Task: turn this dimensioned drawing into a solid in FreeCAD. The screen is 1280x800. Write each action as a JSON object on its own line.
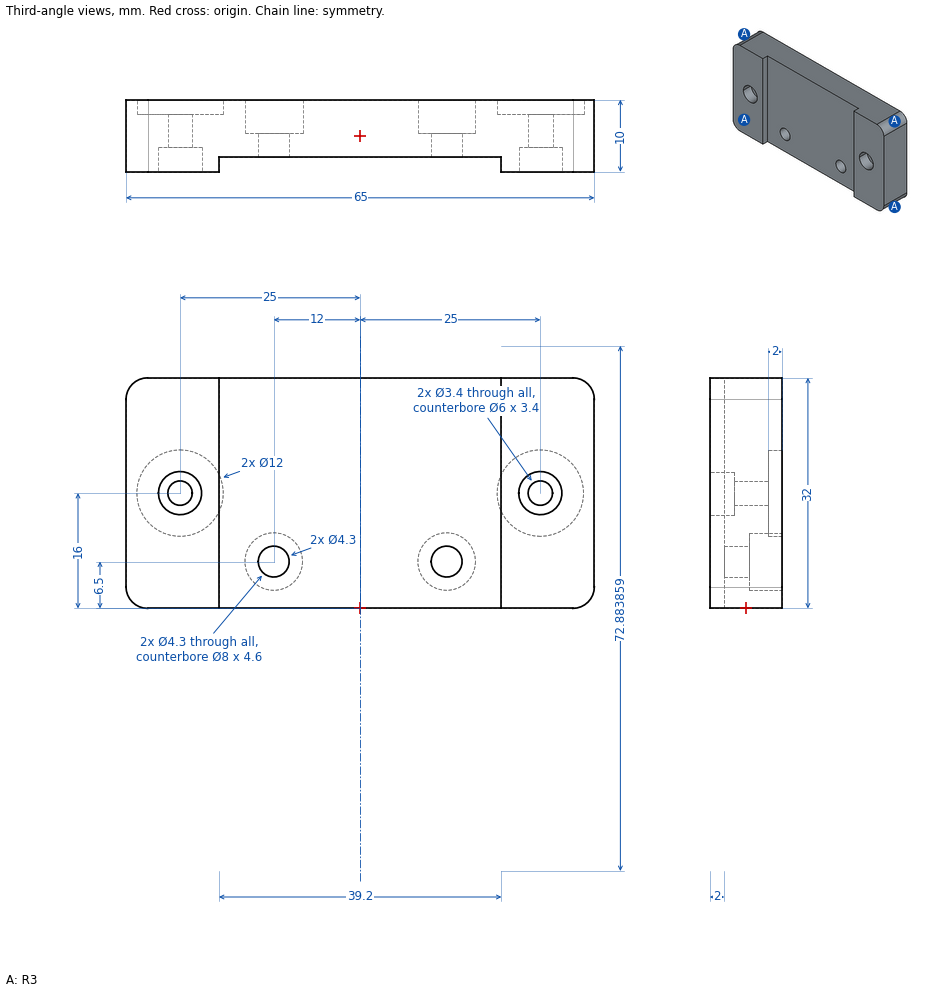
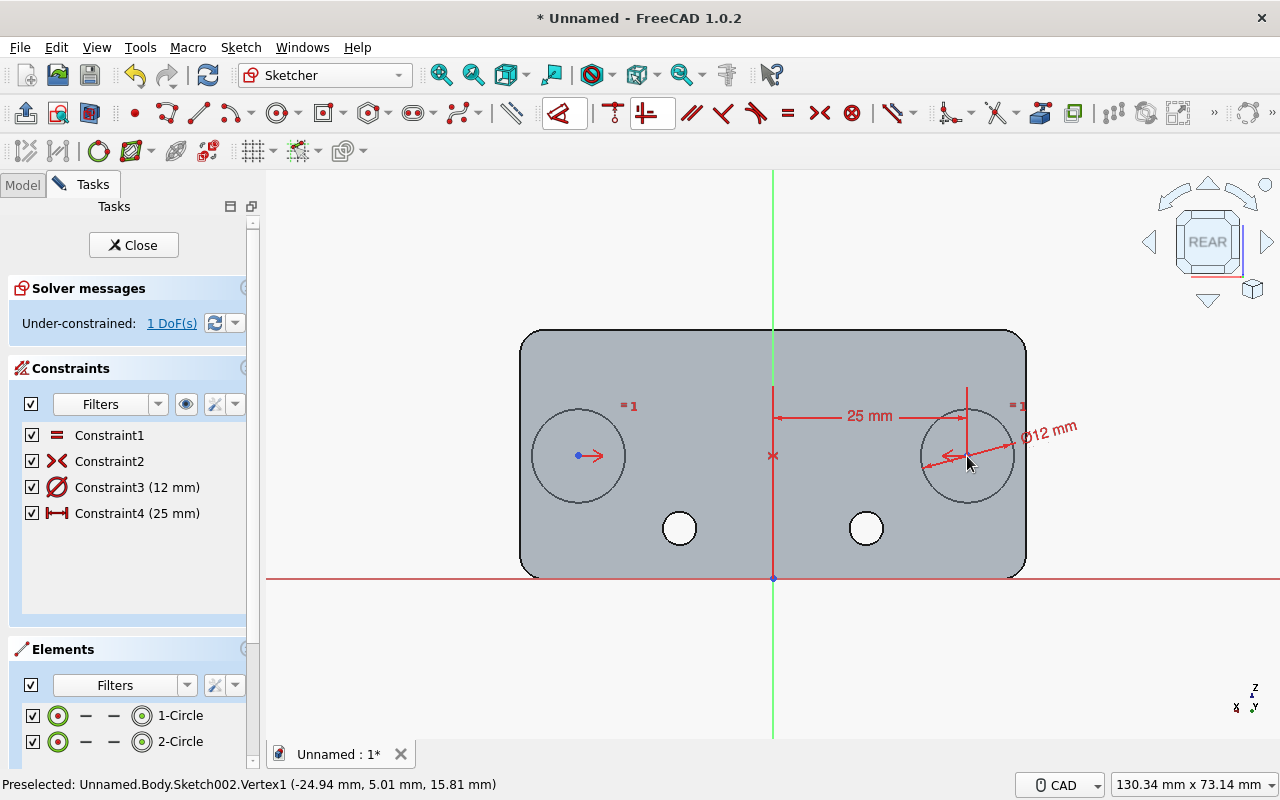
{"action": "left_click", "coordinate": [967, 456]}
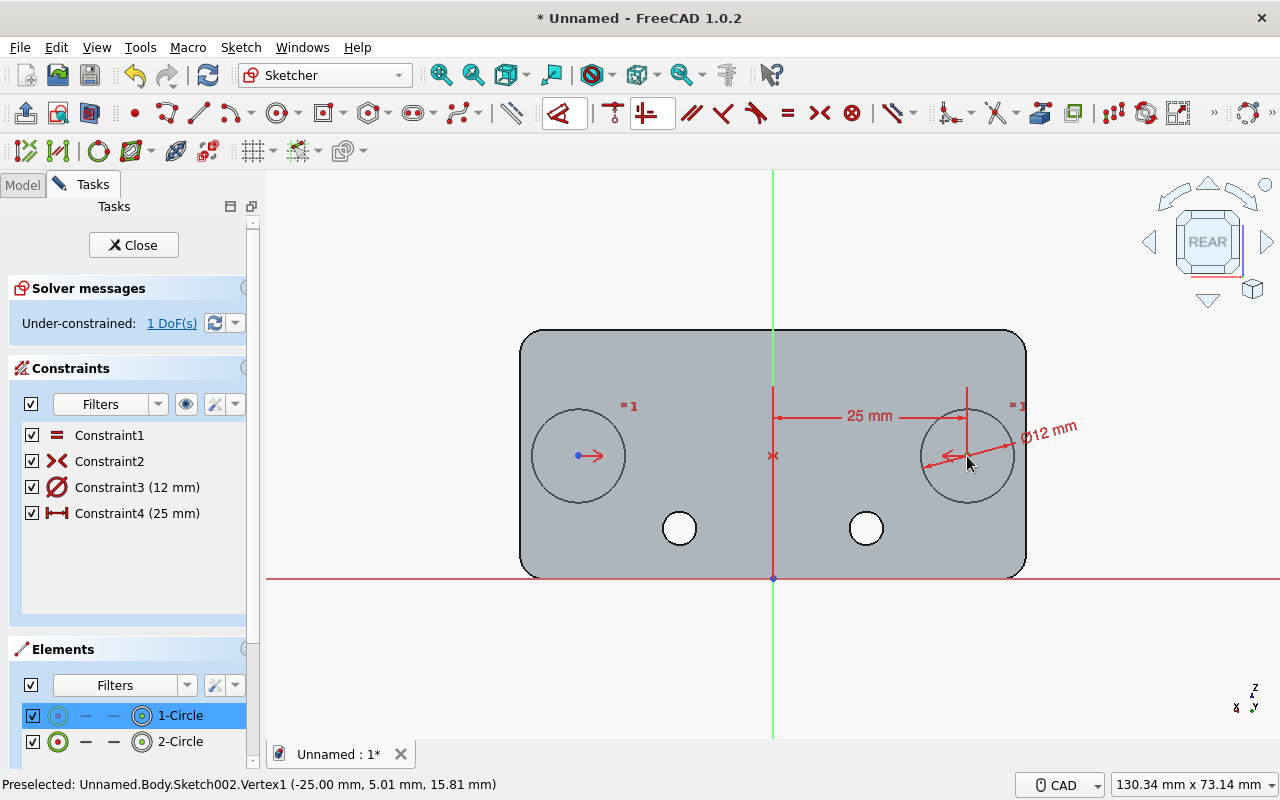
{"action": "left_click", "coordinate": [582, 114]}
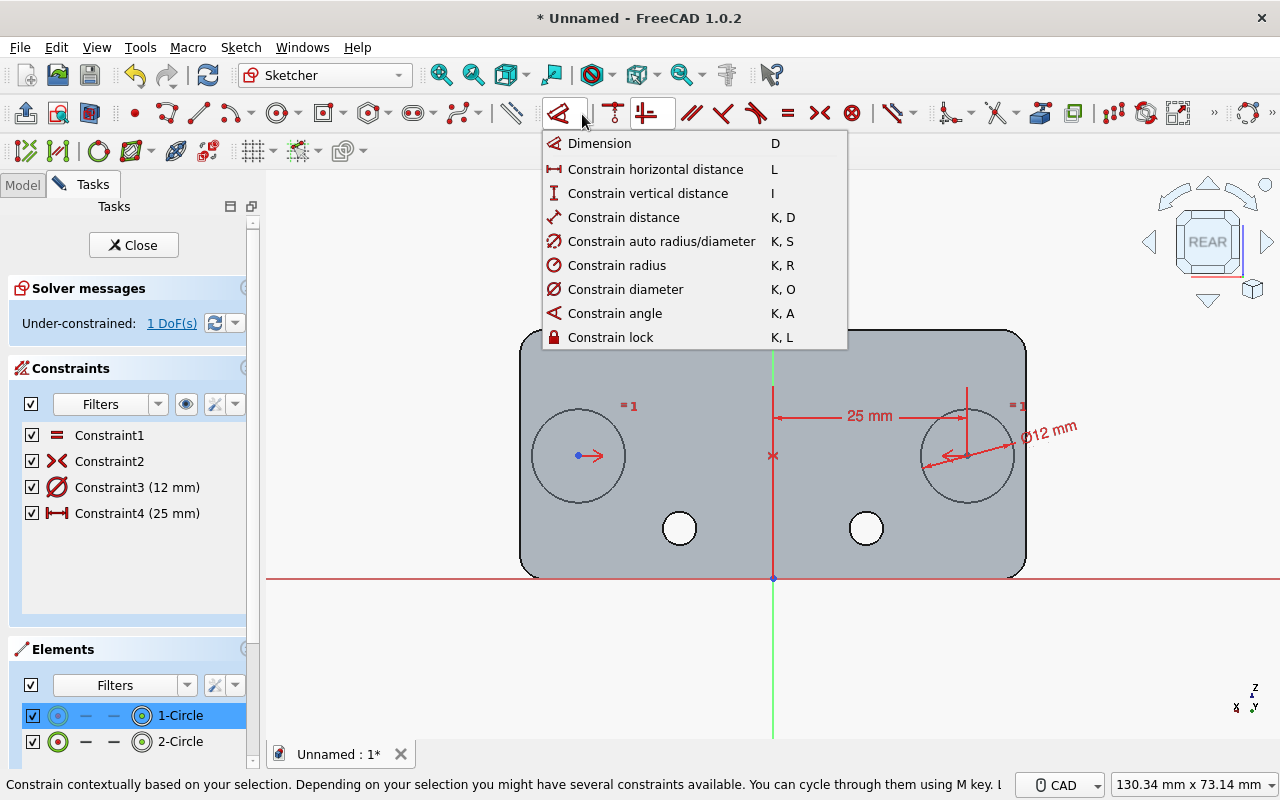
{"action": "left_click", "coordinate": [695, 193]}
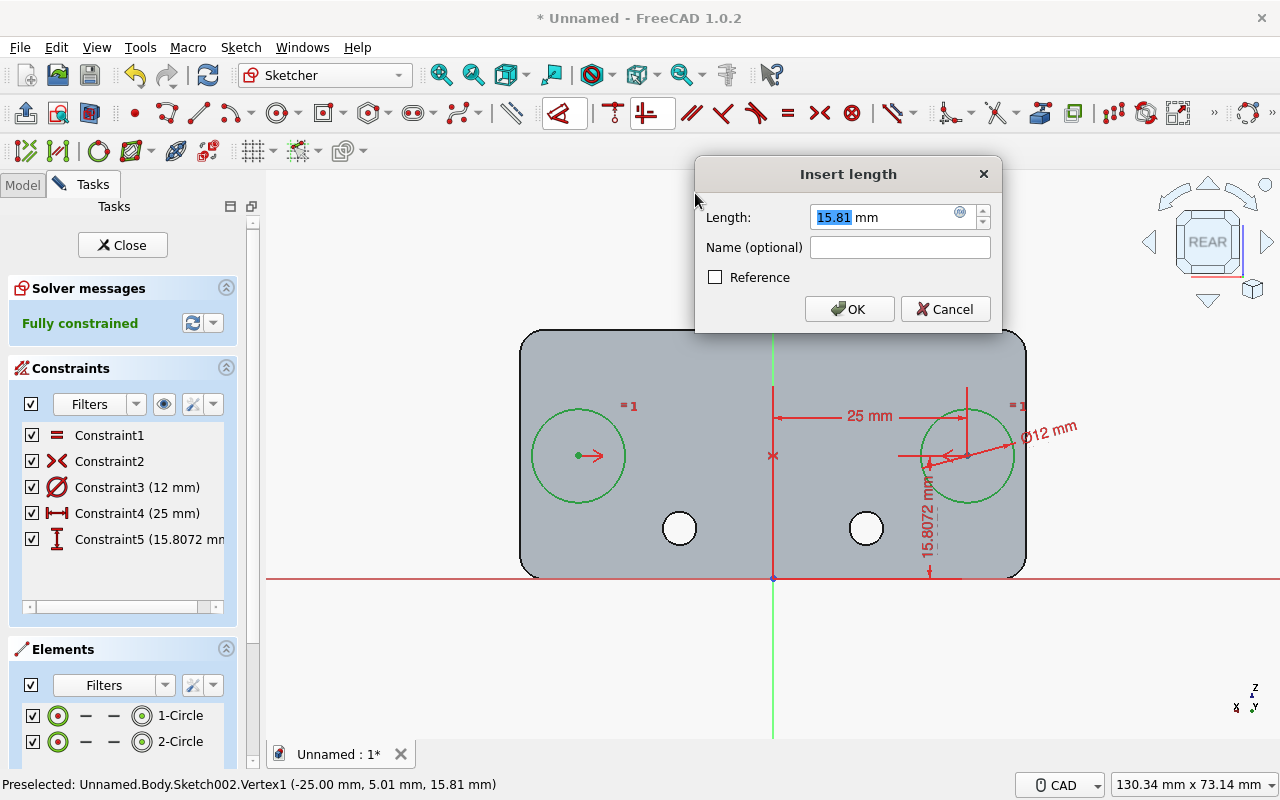
{"action": "type", "text": "16"}
{"action": "key", "text": "Return"}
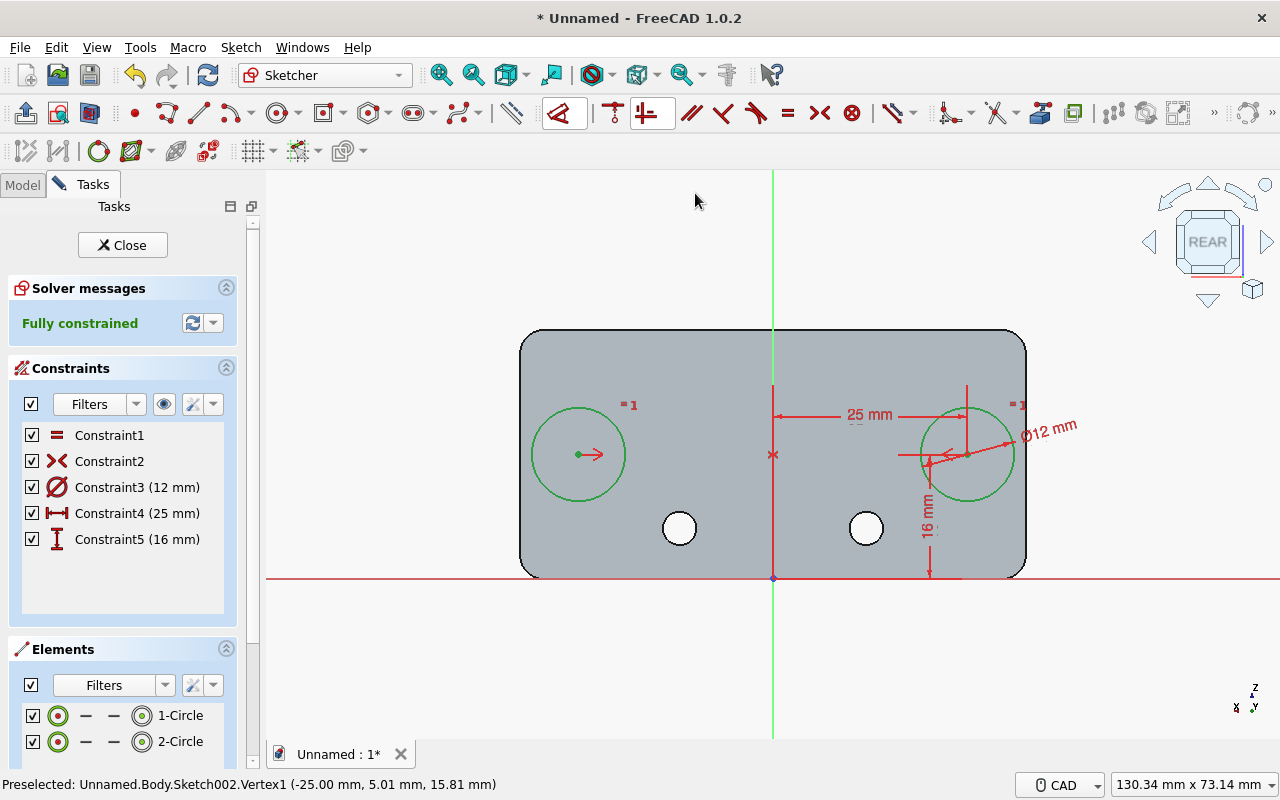
{"action": "left_click", "coordinate": [123, 245]}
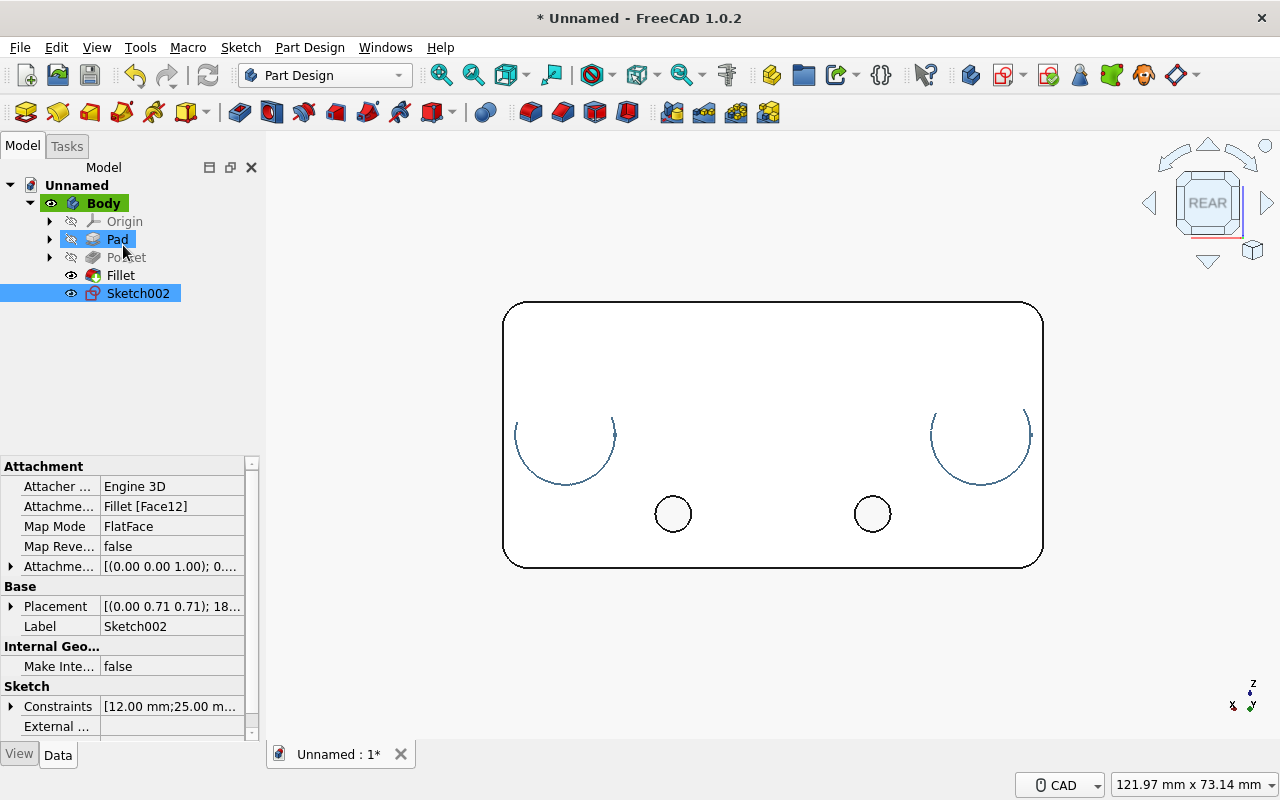
{"action": "left_click", "coordinate": [240, 112]}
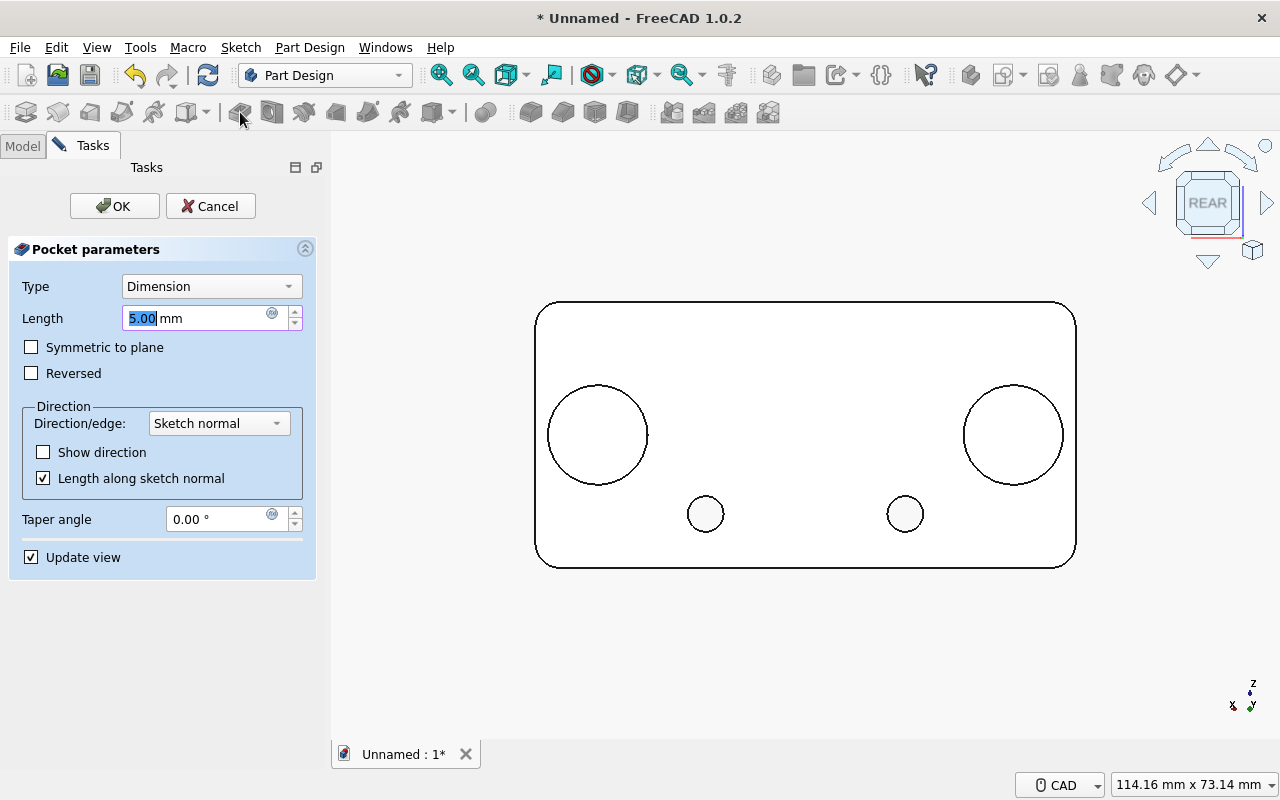
{"action": "type", "text": "2"}
{"action": "key", "text": "Tab"}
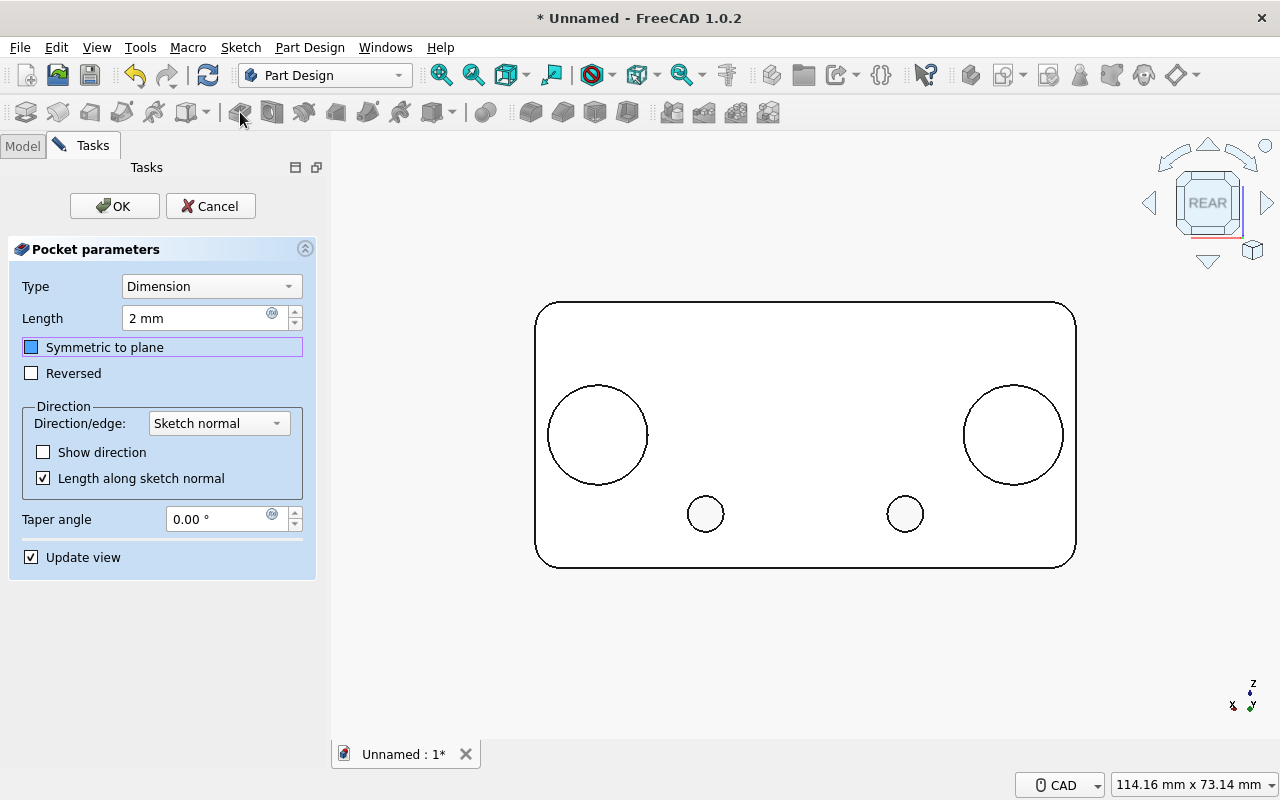
{"action": "left_click", "coordinate": [115, 206]}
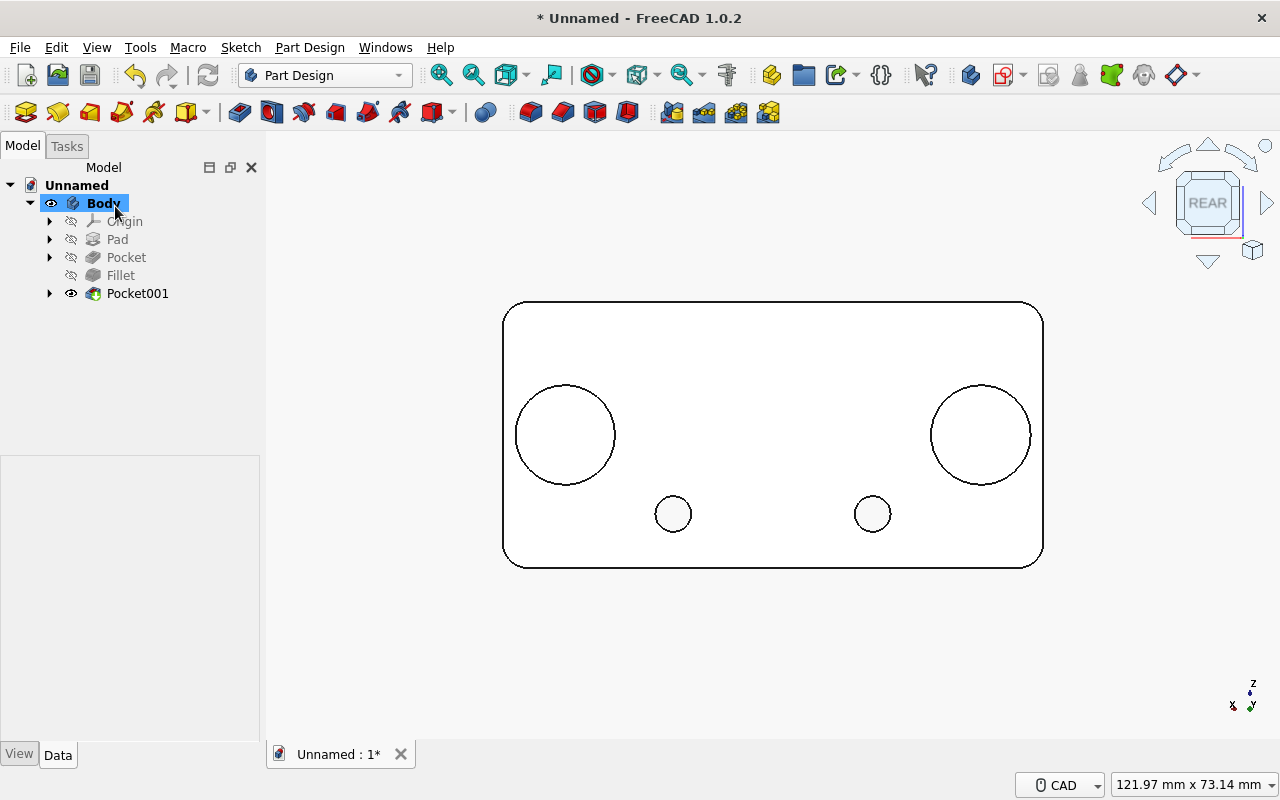
{"action": "key", "text": "0"}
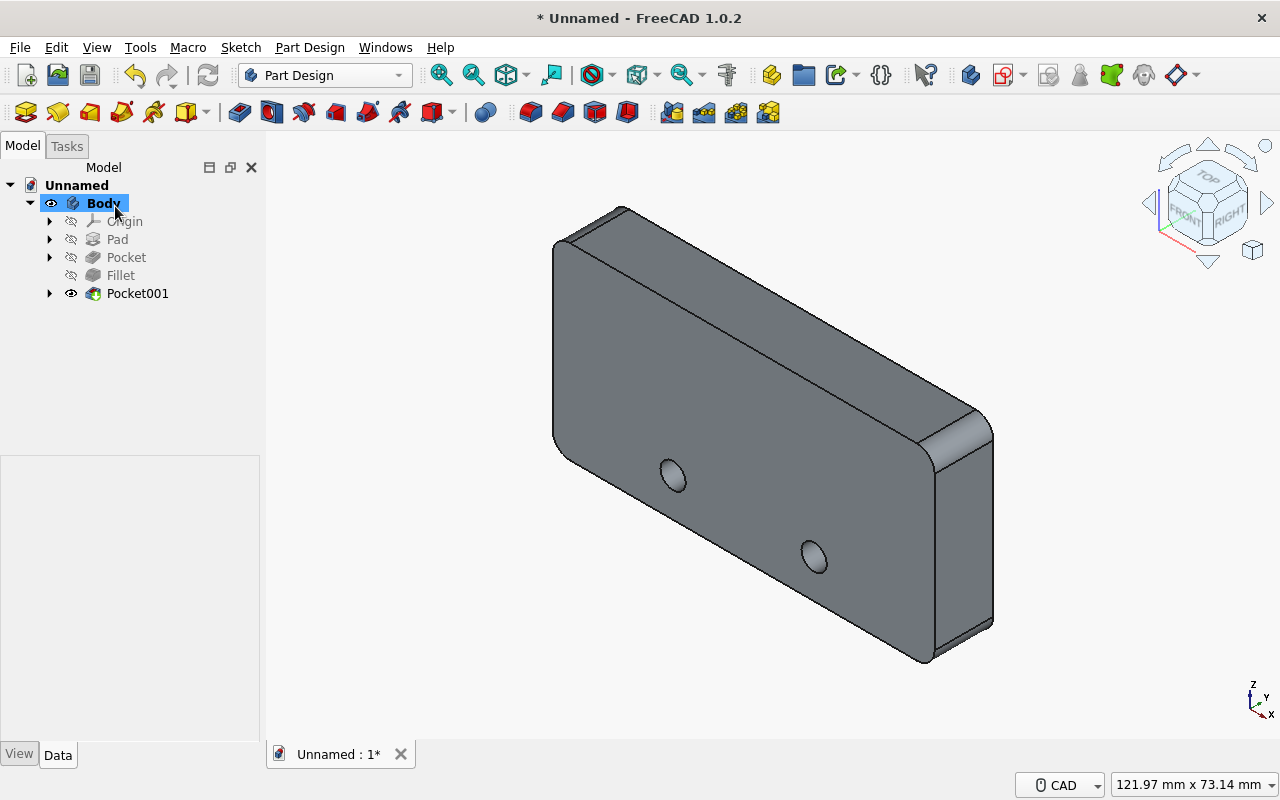
{"action": "left_click", "coordinate": [744, 451]}